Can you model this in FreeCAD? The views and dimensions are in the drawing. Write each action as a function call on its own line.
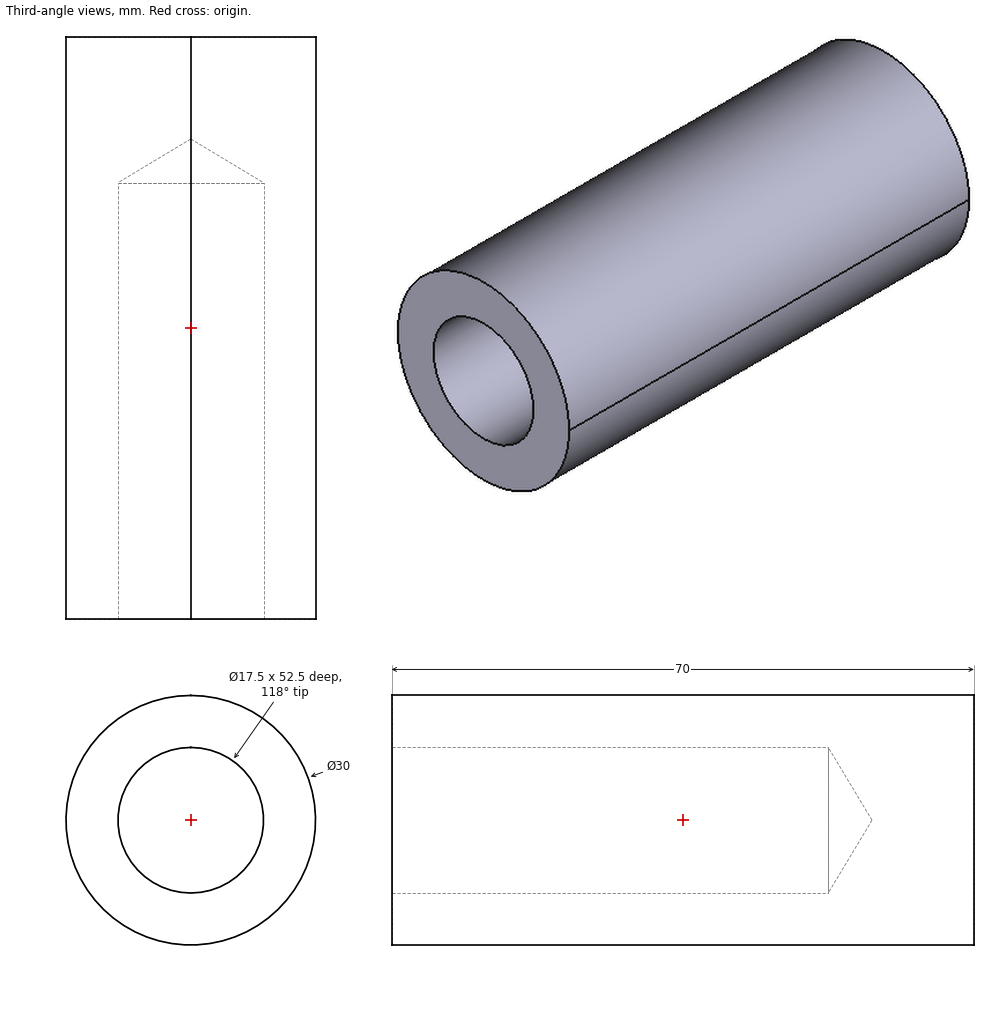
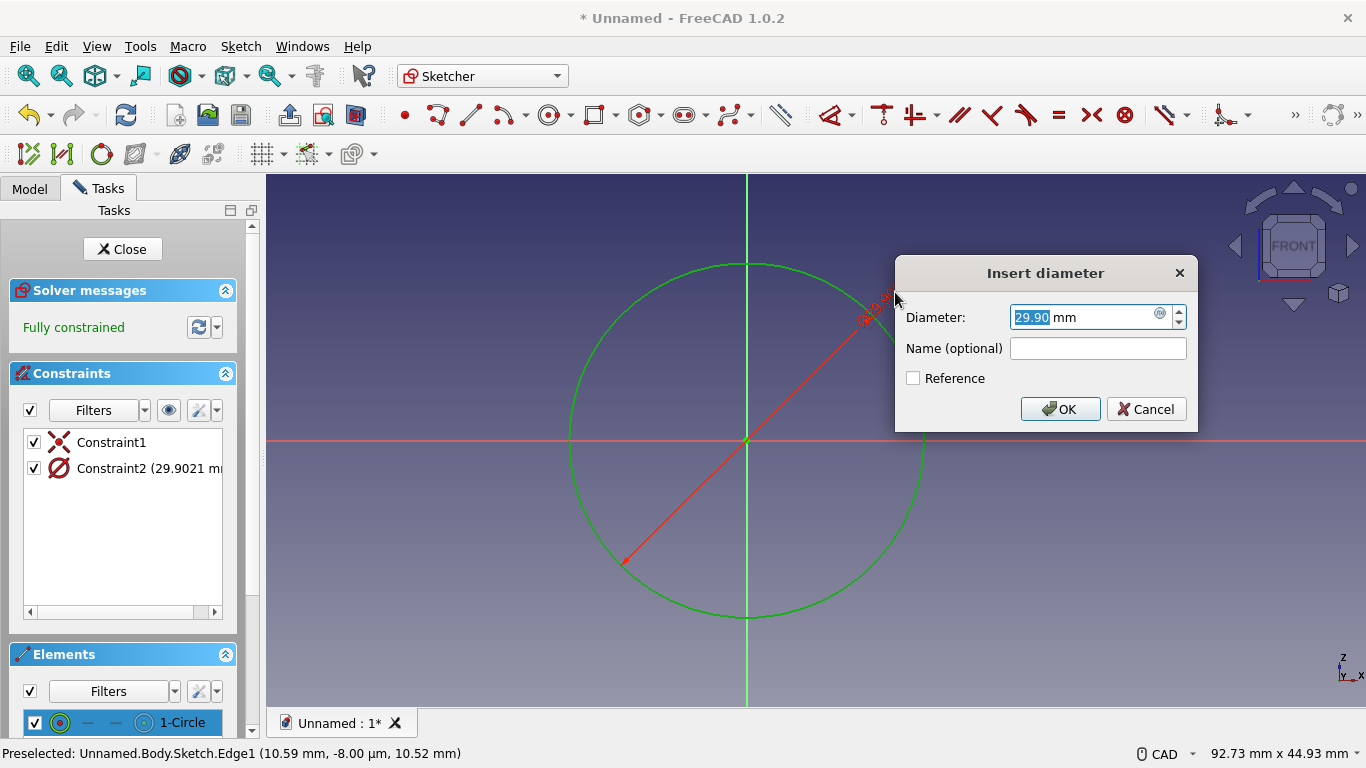
text(30)
key(Return)
key(Escape)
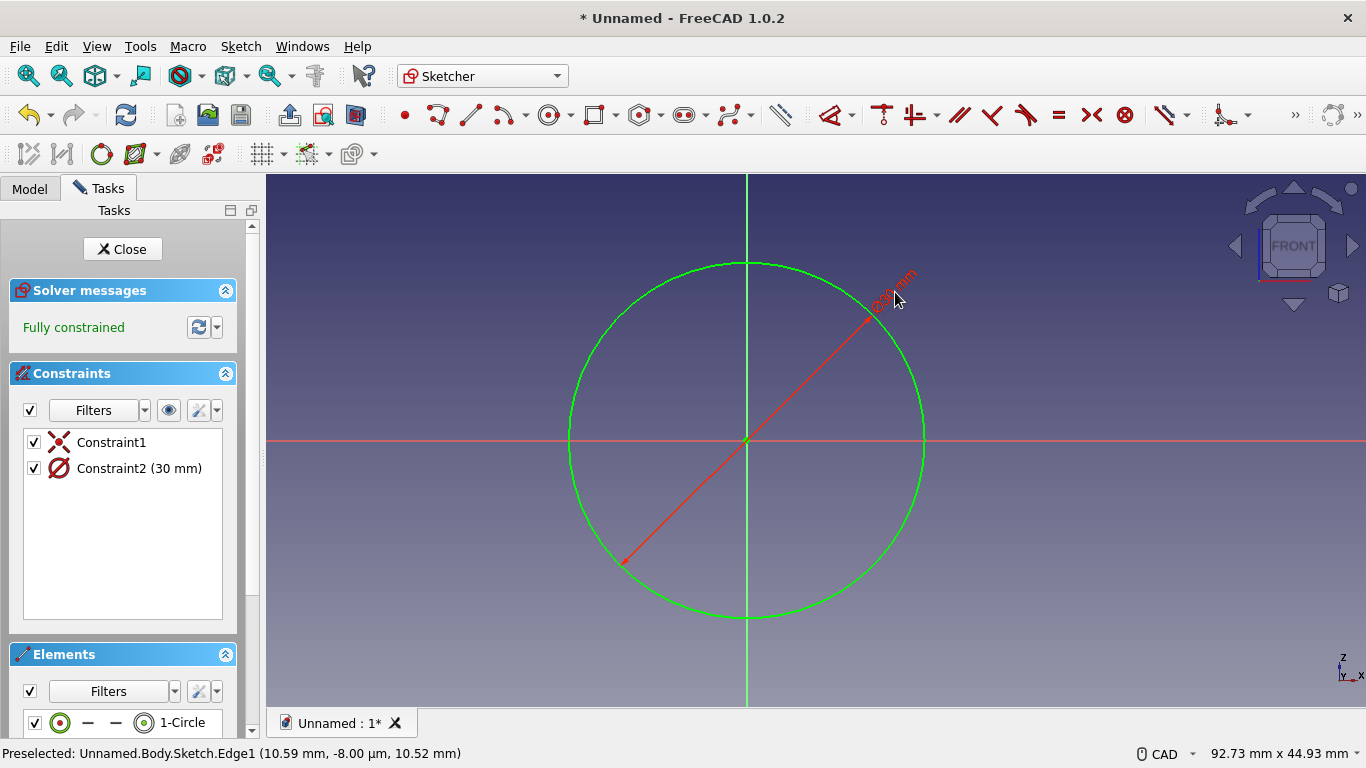
click(123, 249)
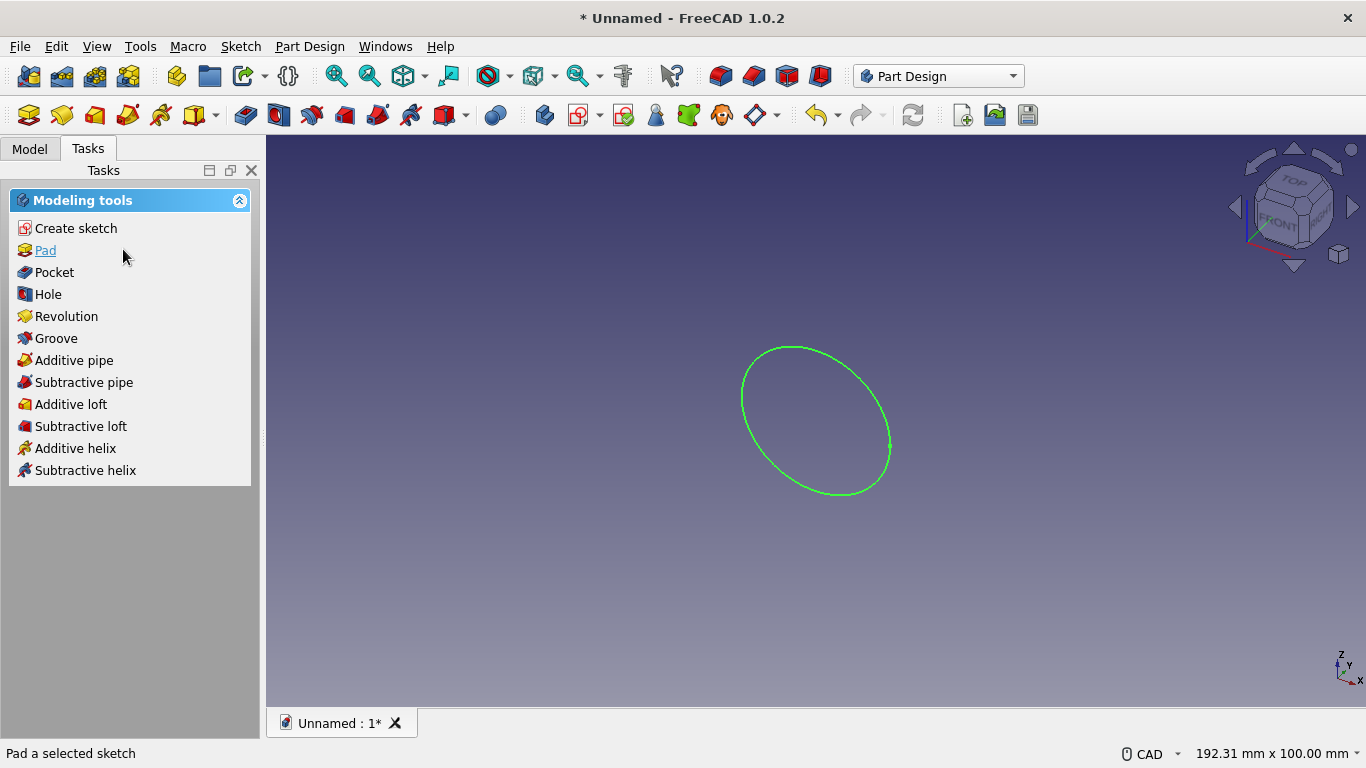
click(29, 116)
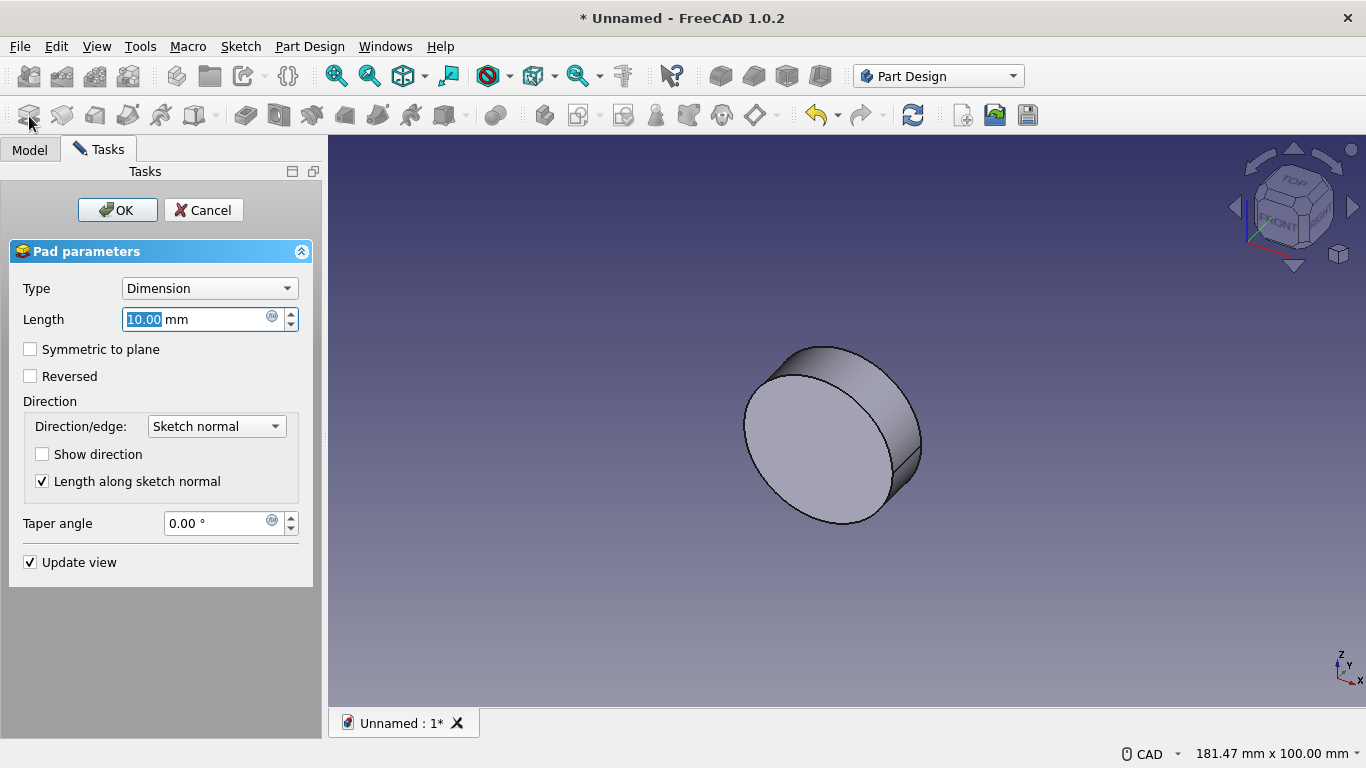
text(70)
key(Tab)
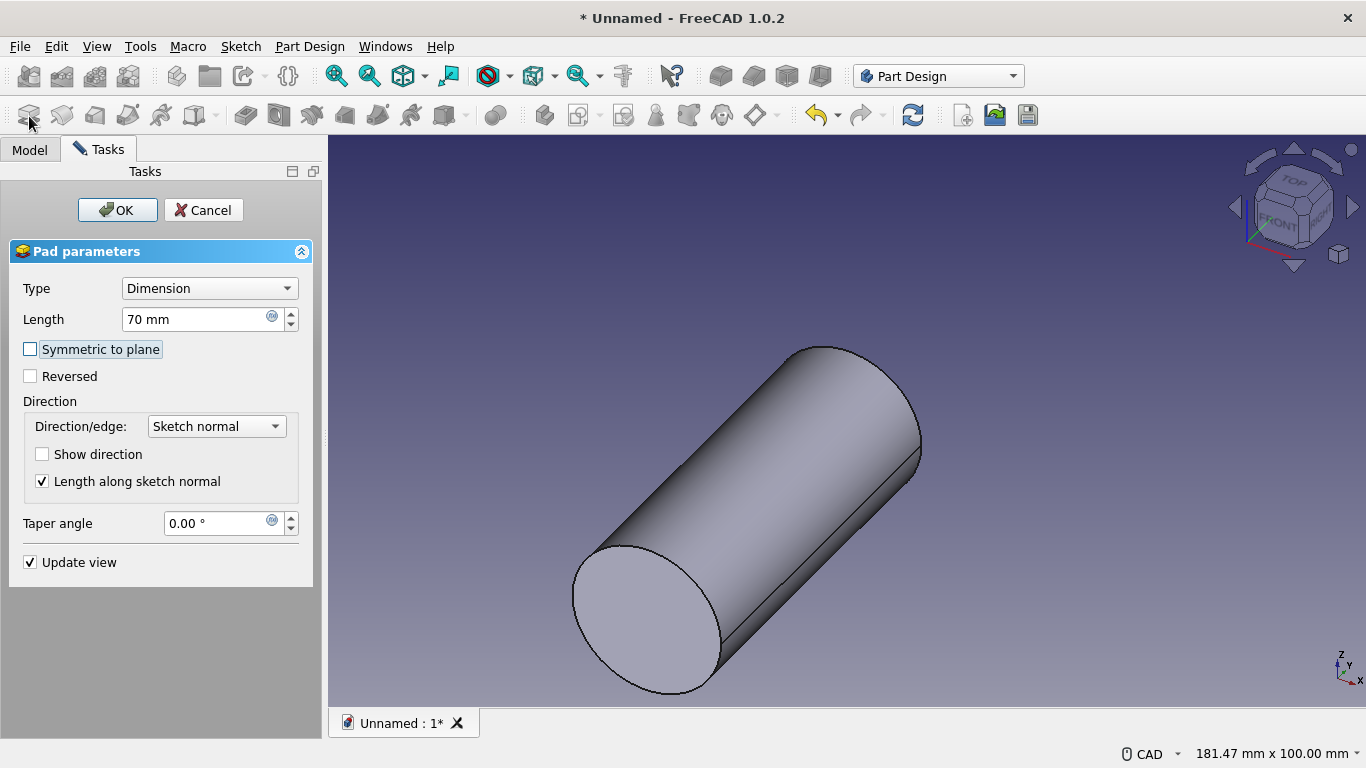
click(31, 349)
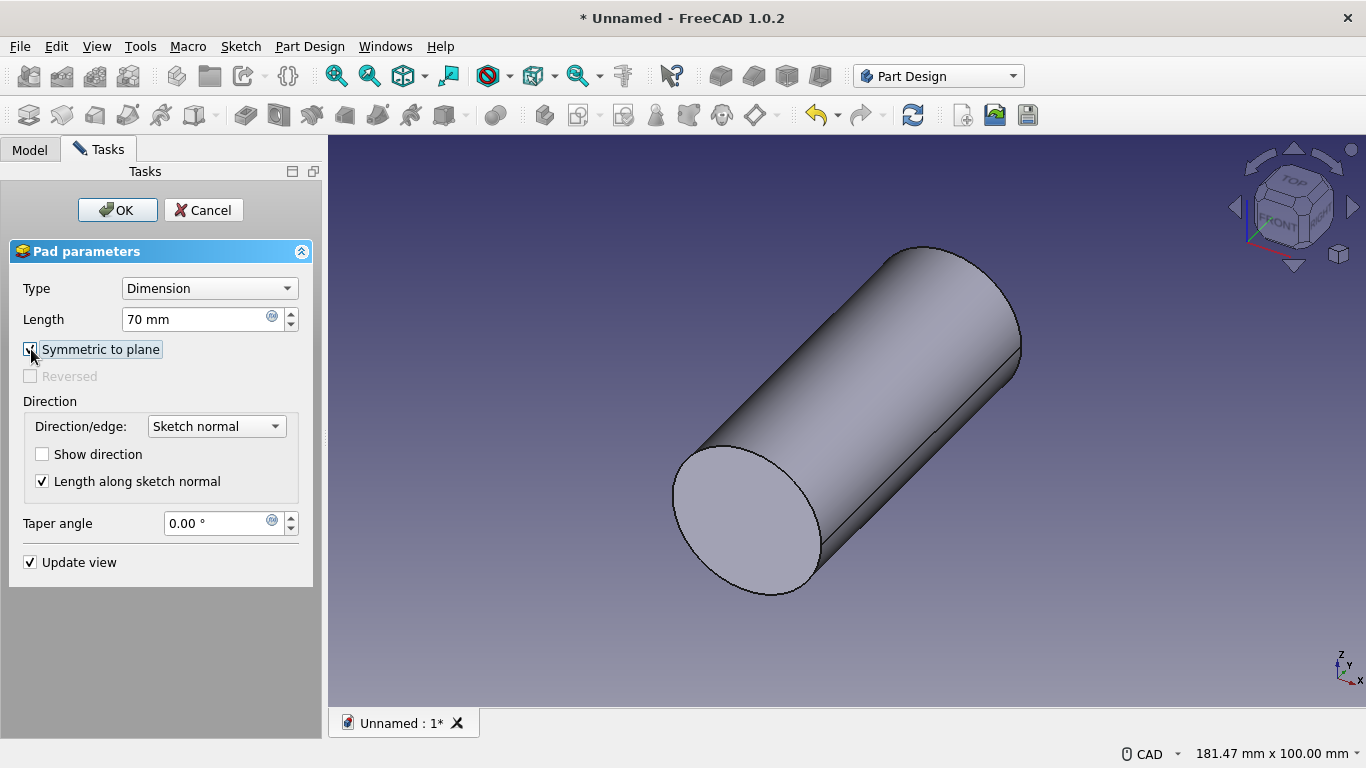
click(118, 210)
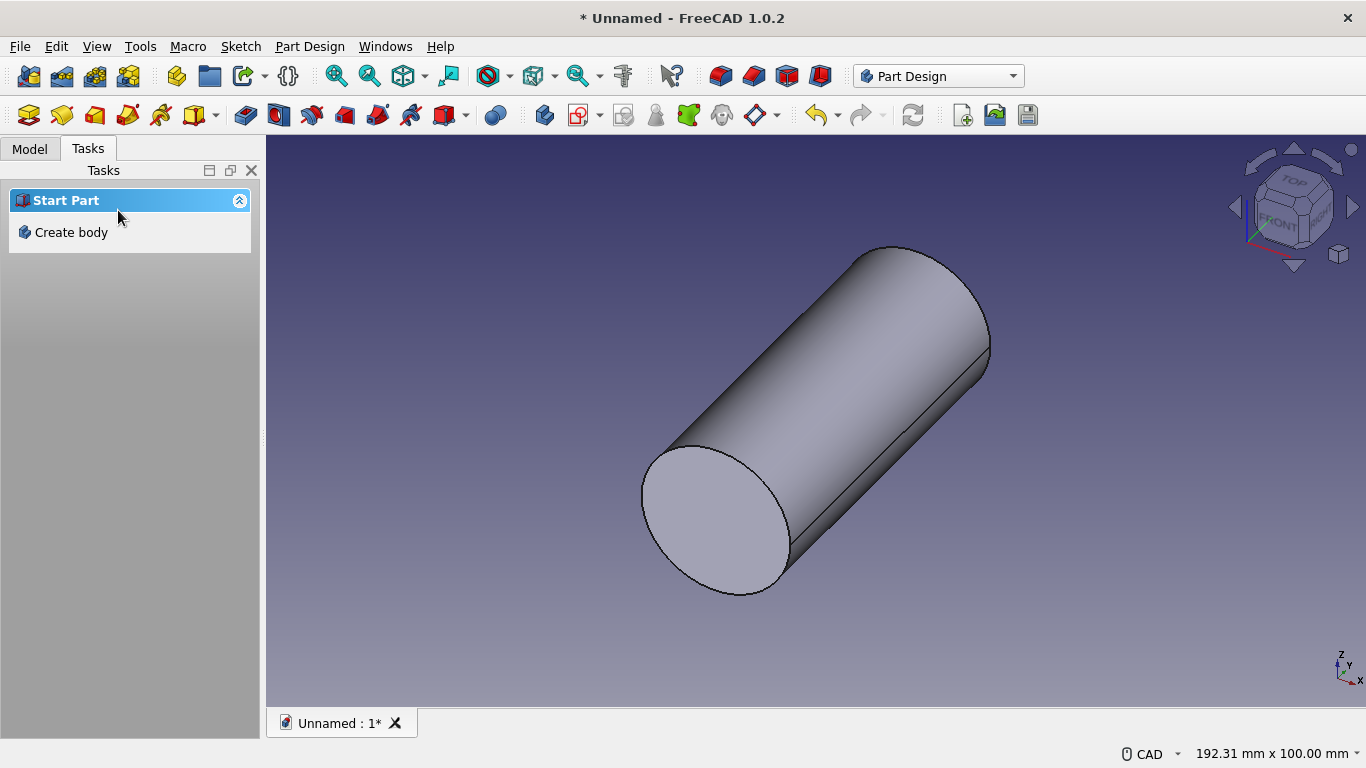
click(716, 519)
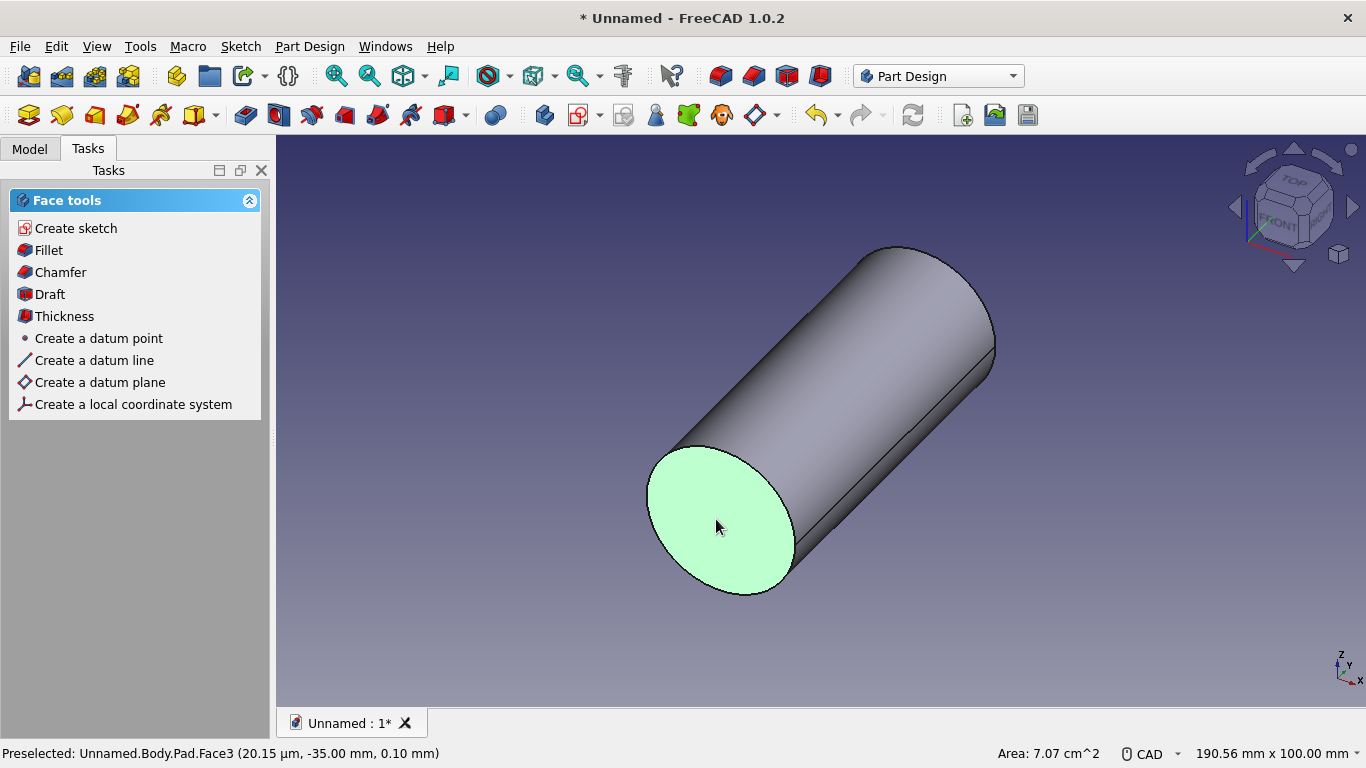
click(578, 116)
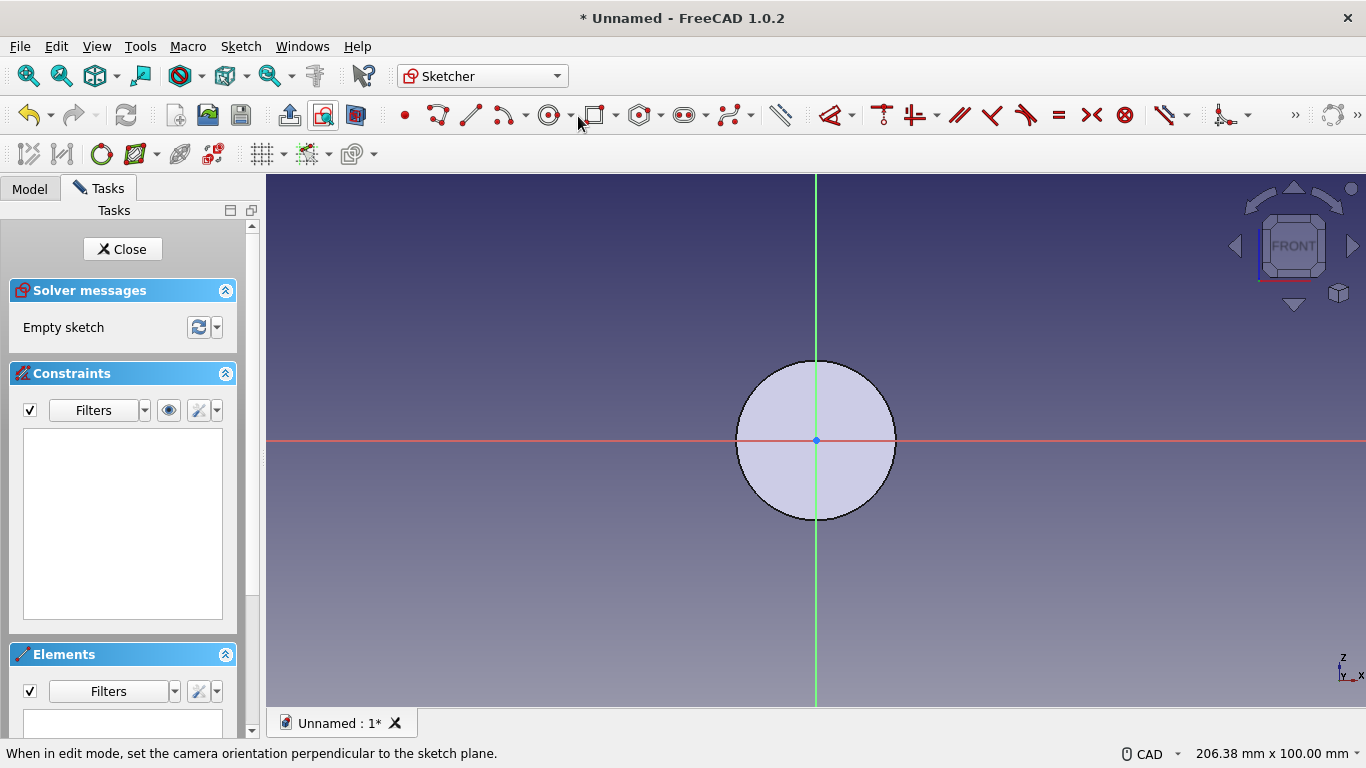
scroll(846, 440, up, 6)